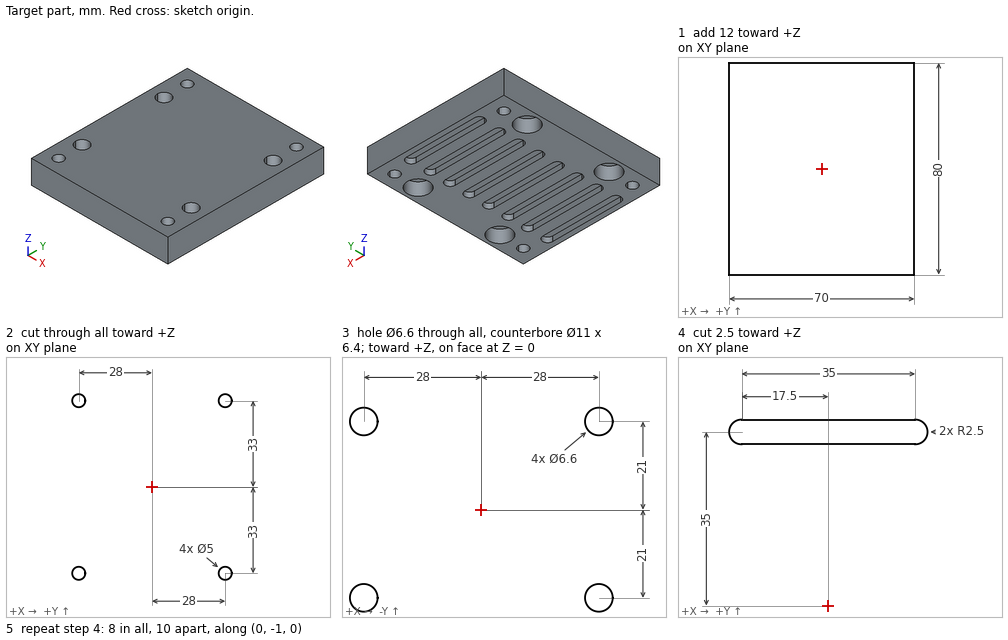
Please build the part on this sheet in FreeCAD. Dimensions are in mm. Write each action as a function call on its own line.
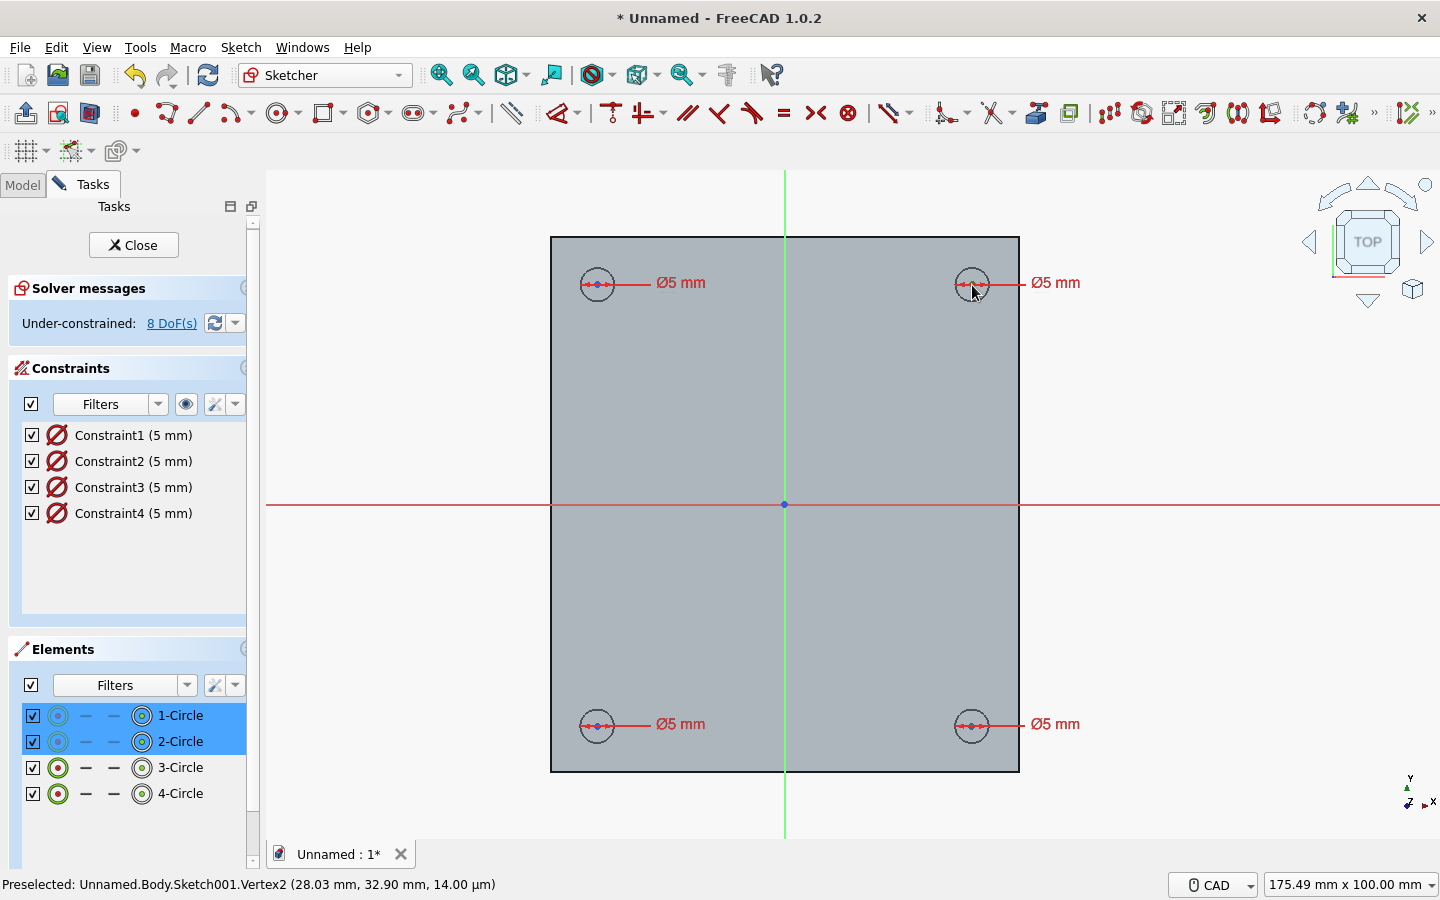
click(666, 114)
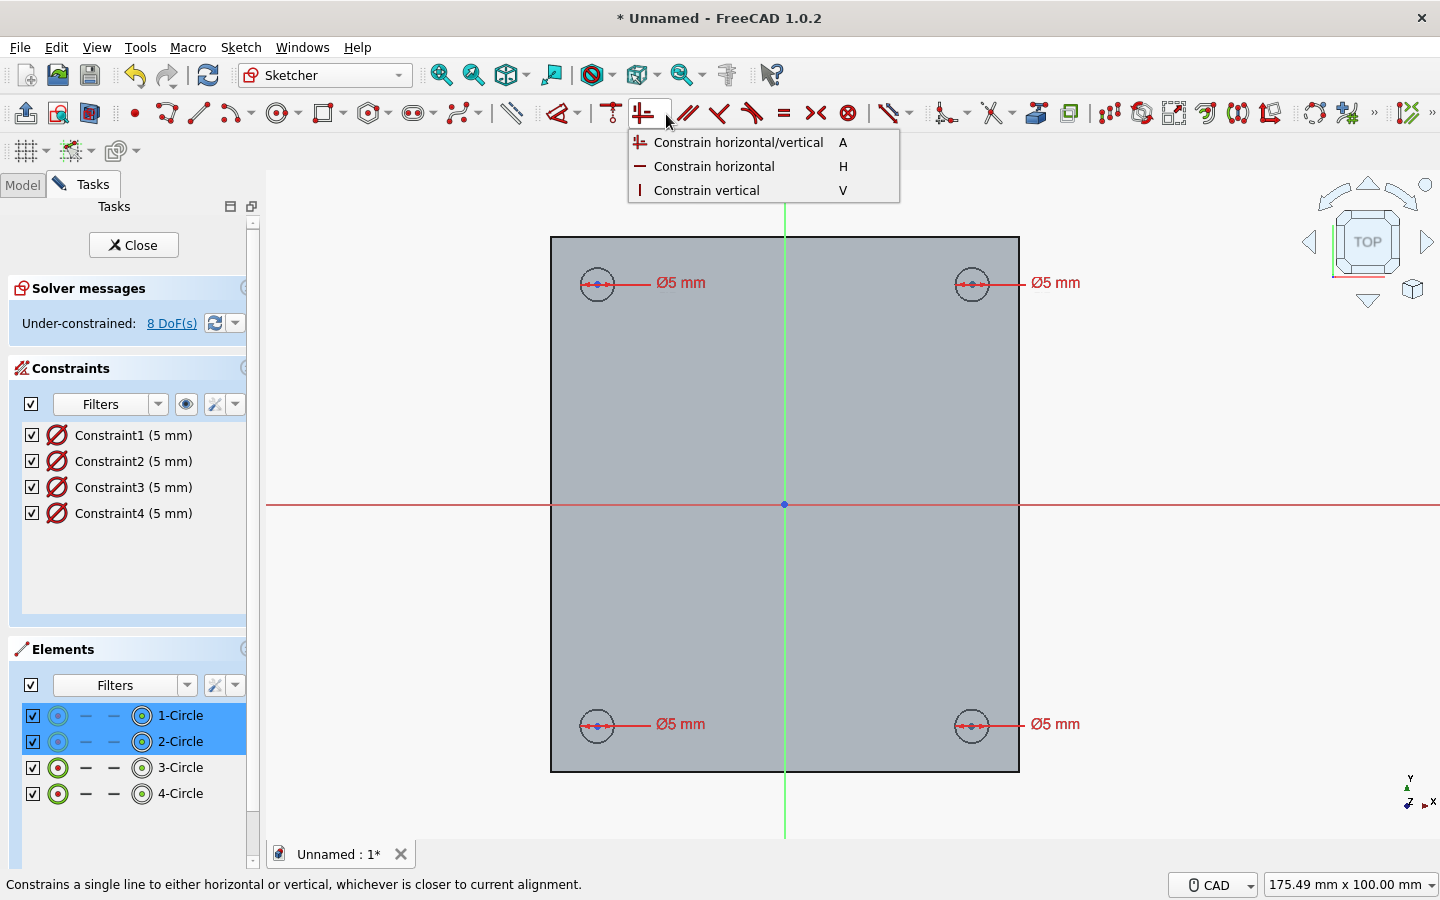
click(764, 190)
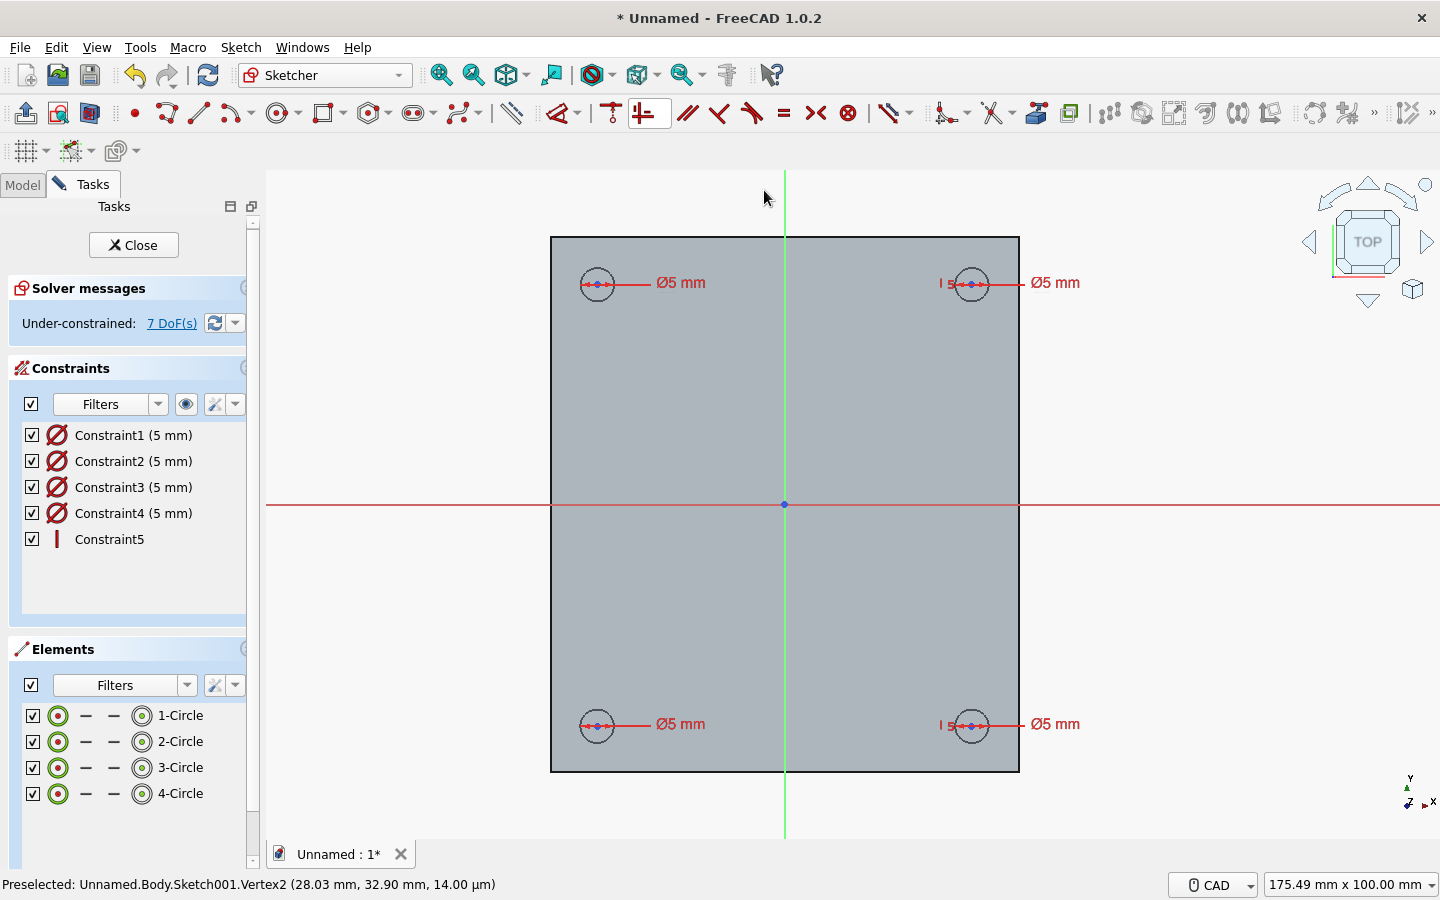
click(972, 285)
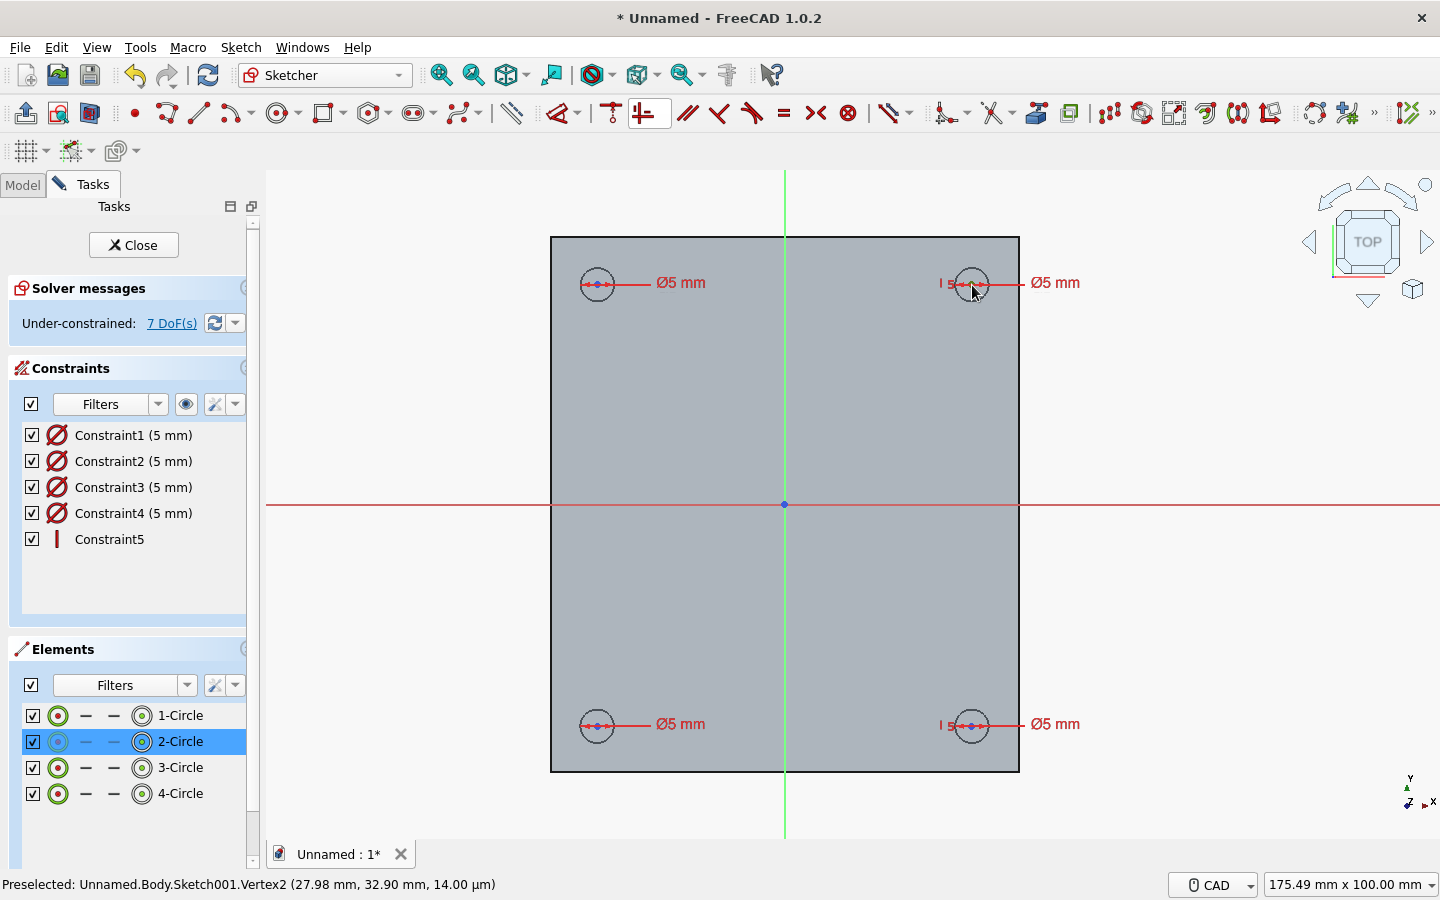
click(597, 285)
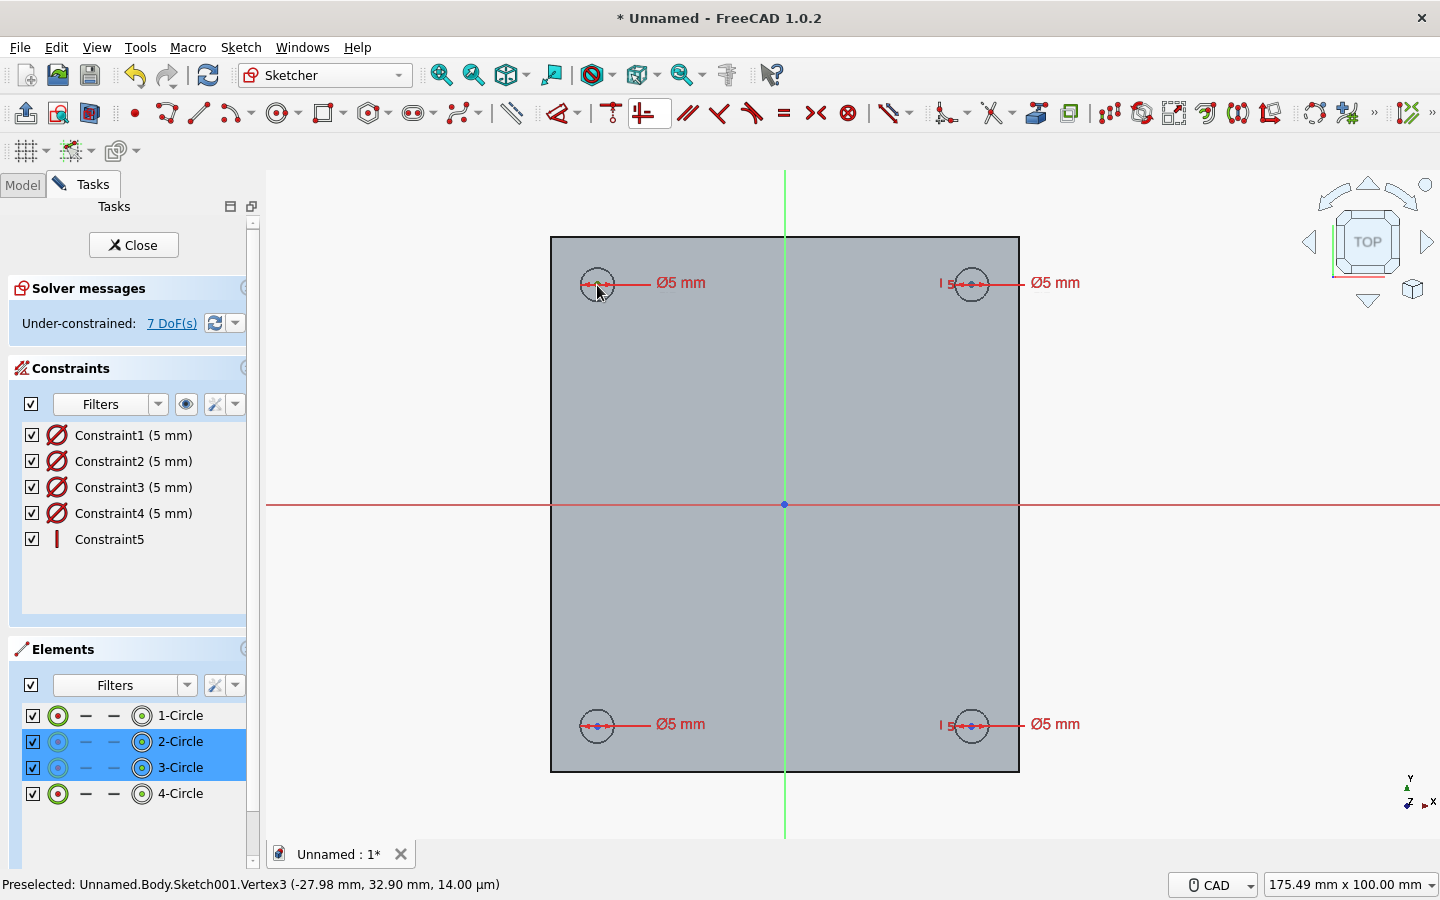
key(h)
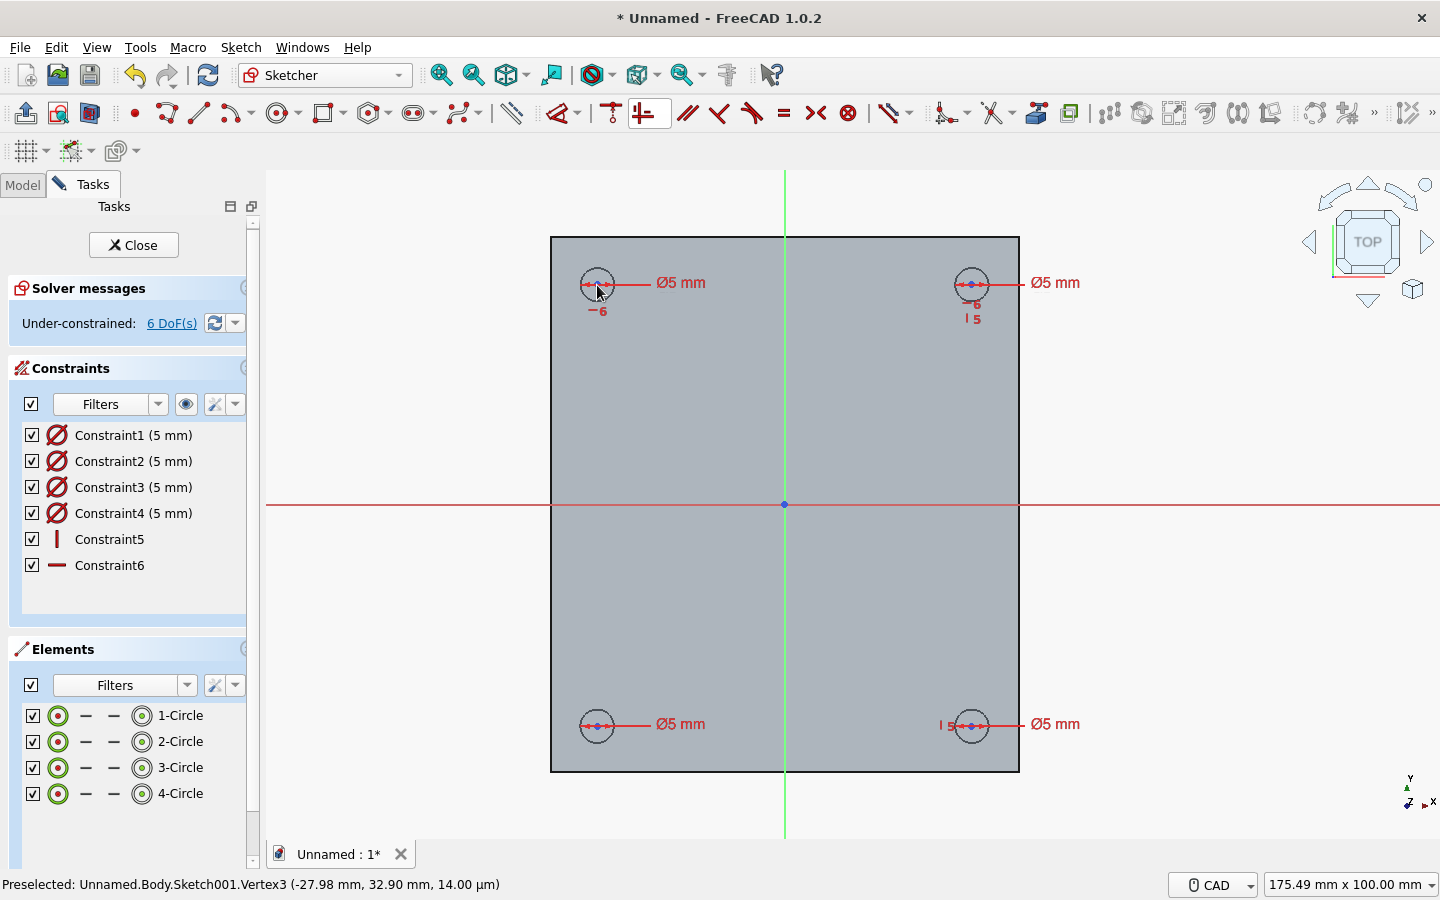
click(597, 285)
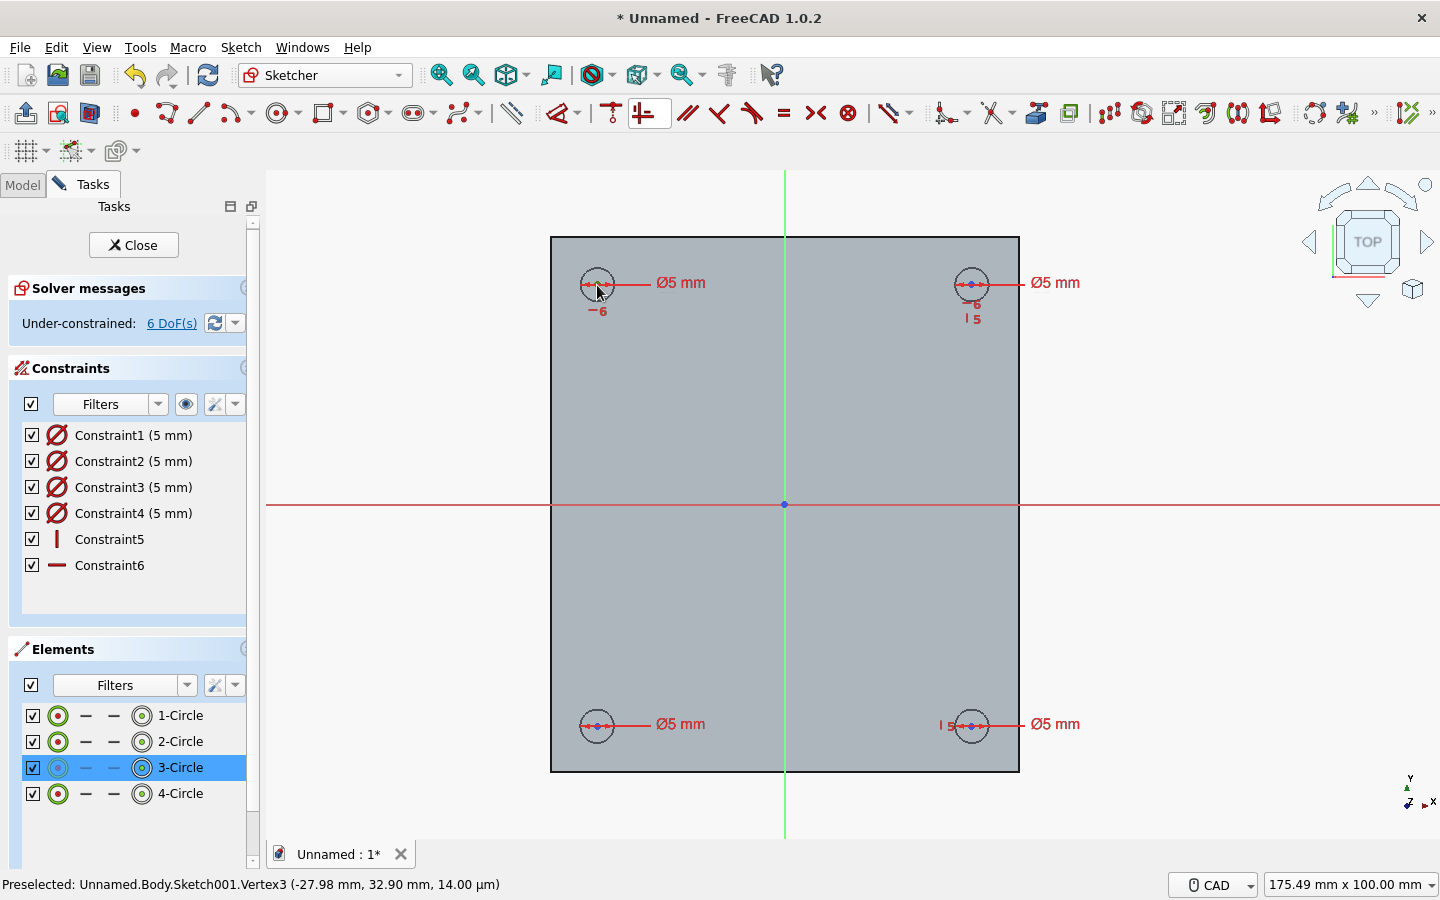
click(597, 726)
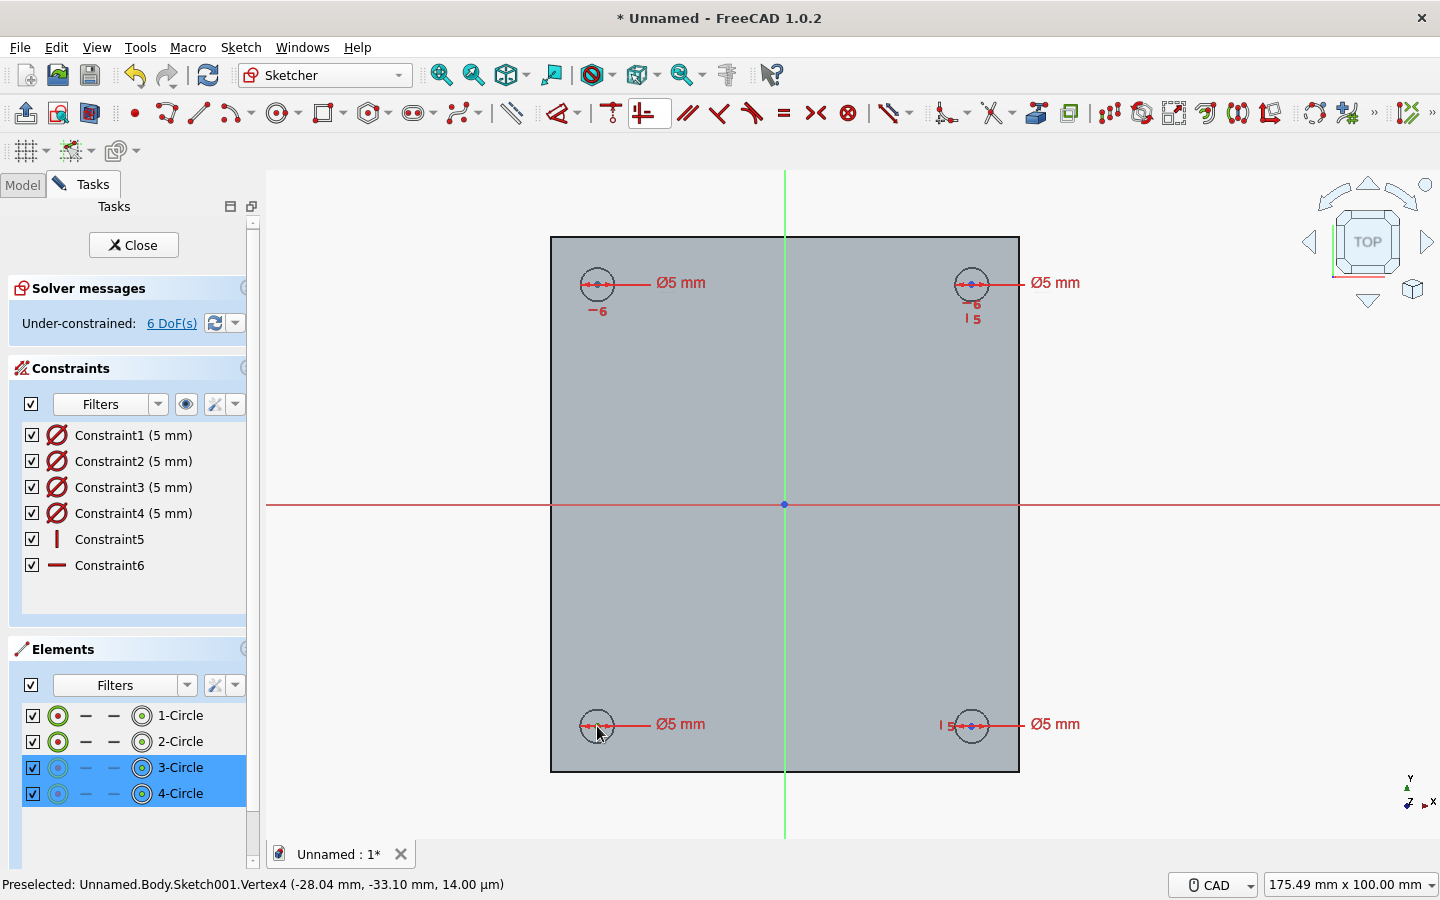
click(666, 114)